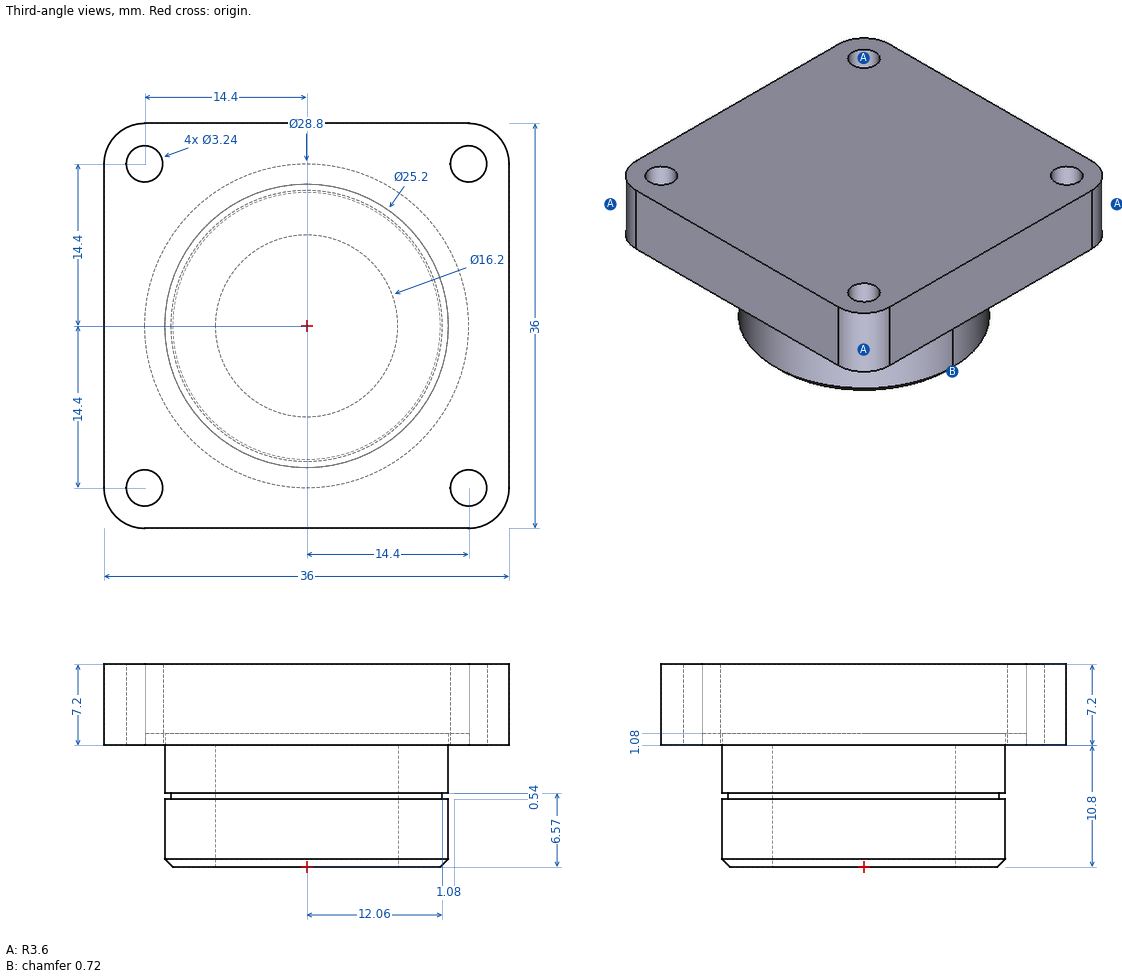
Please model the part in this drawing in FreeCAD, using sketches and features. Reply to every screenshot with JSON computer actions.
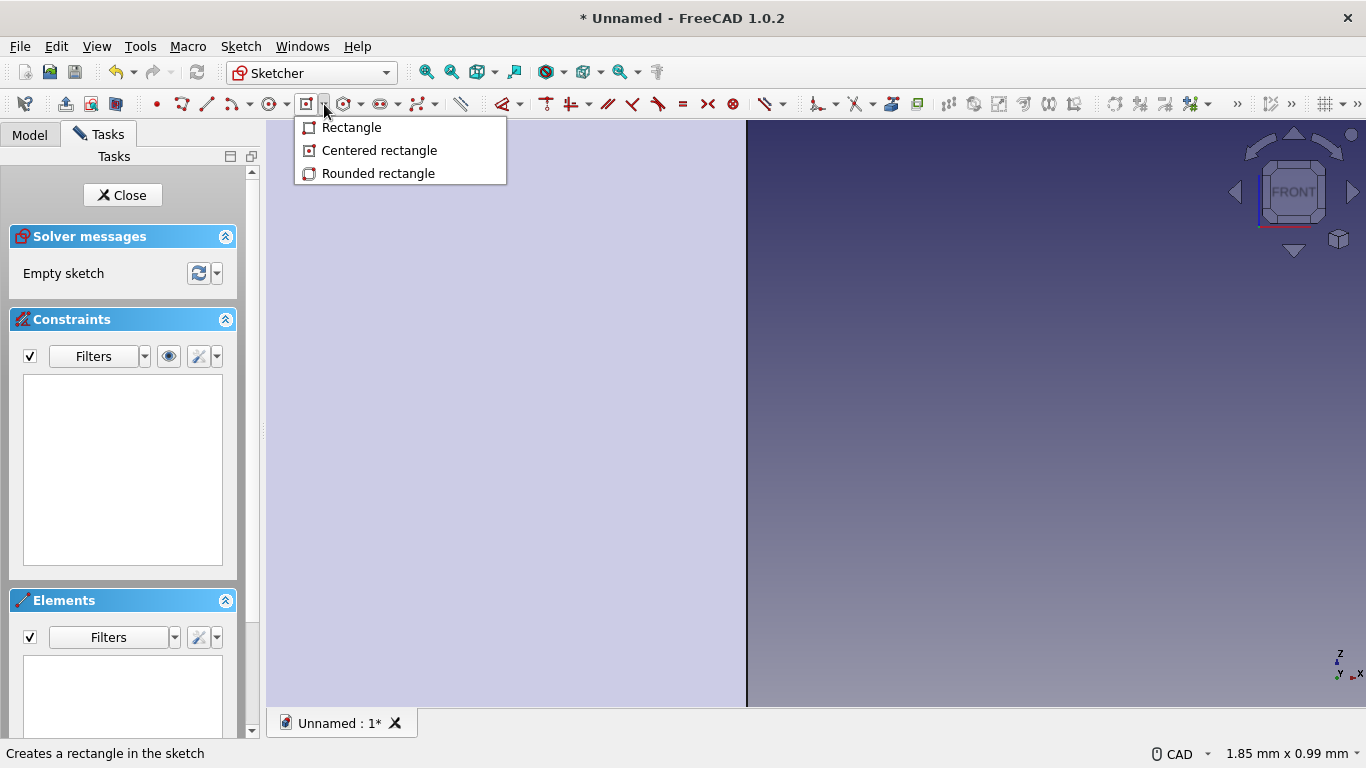
{"action": "left_click", "coordinate": [400, 128]}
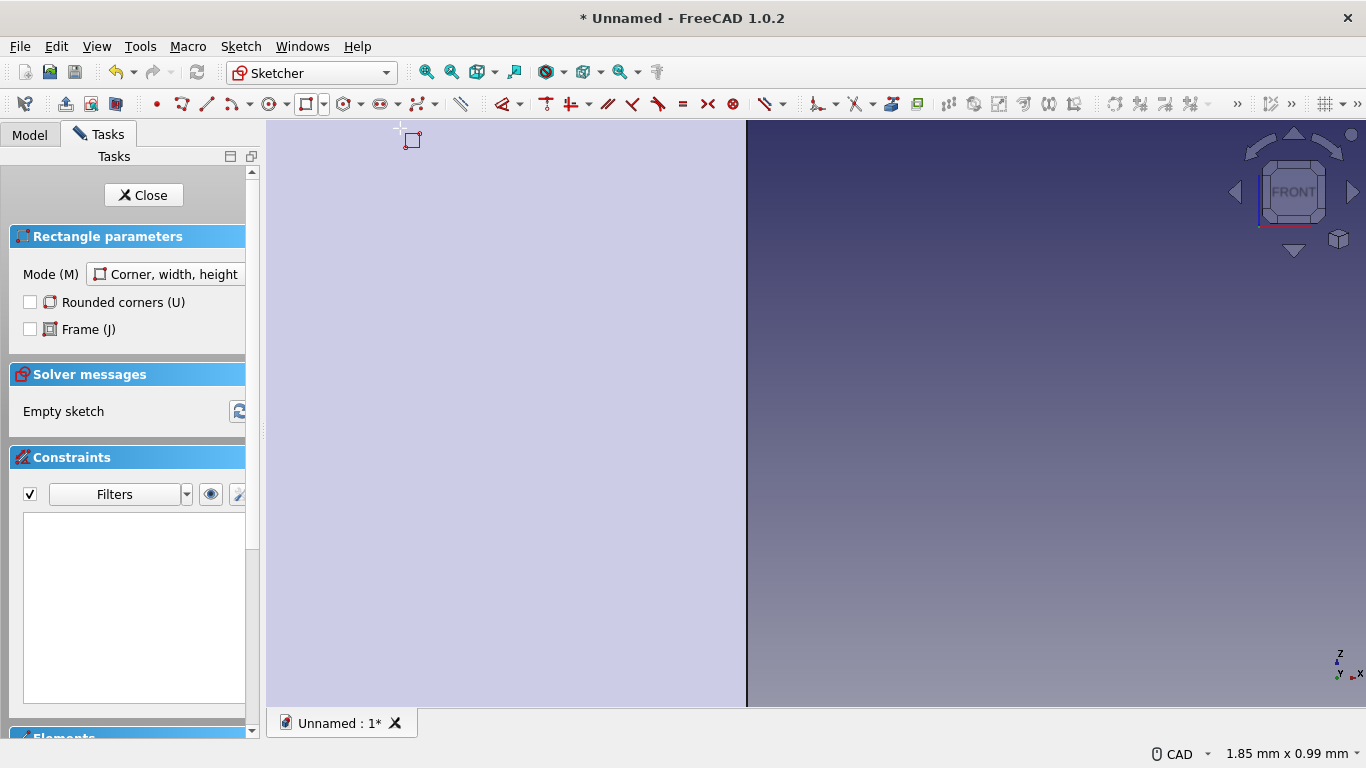
{"action": "left_click", "coordinate": [427, 252]}
{"action": "mouse_move", "coordinate": [1068, 572]}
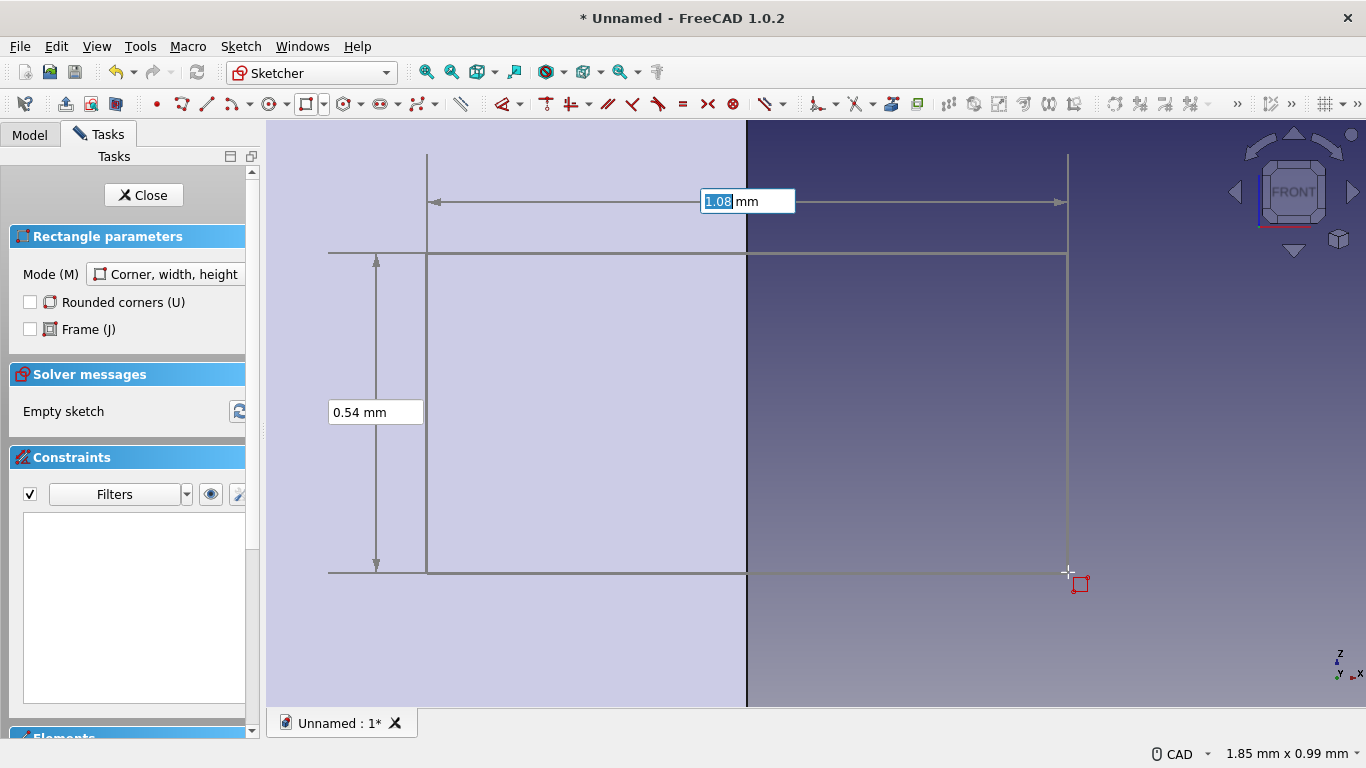
{"action": "type", "text": "1.08"}
{"action": "key", "text": "Tab"}
{"action": "type", "text": "0.54"}
{"action": "key", "text": "Return"}
{"action": "key", "text": "Escape"}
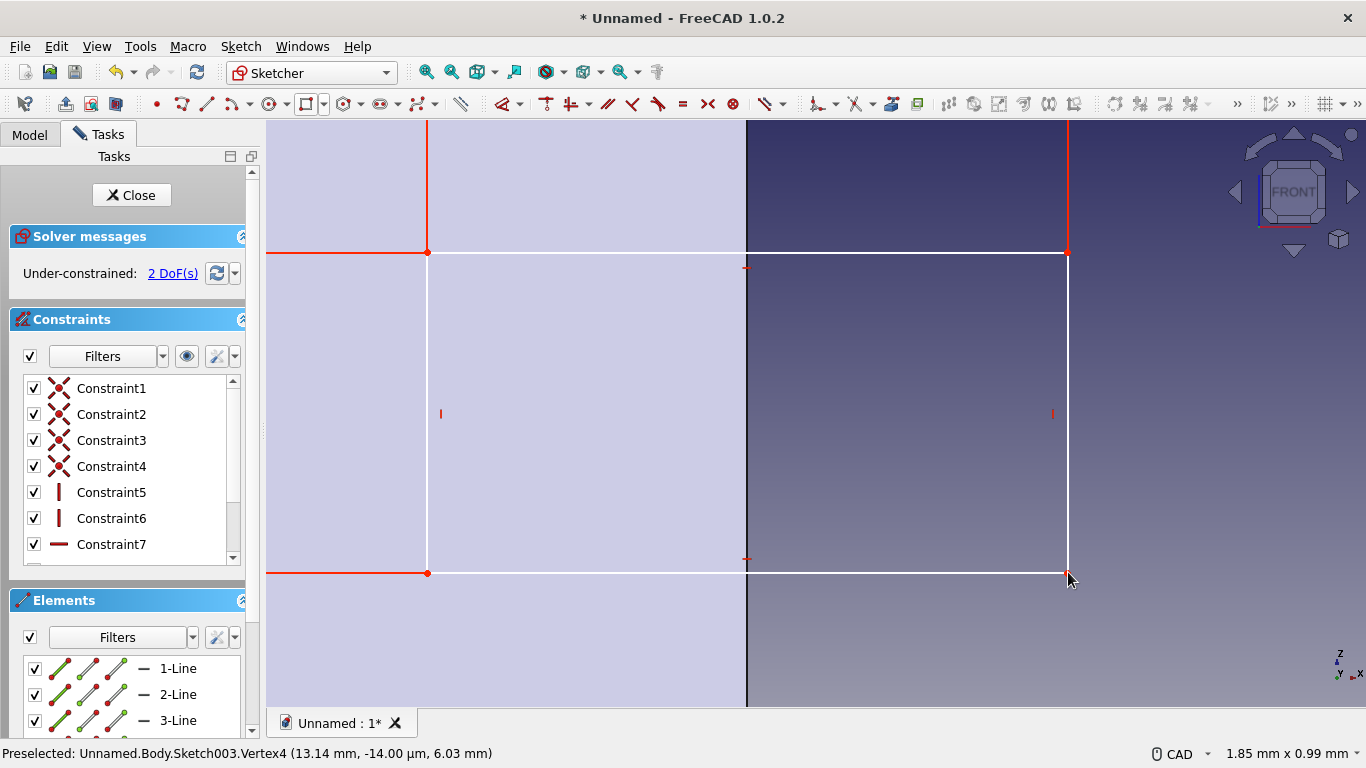
{"action": "left_click", "coordinate": [502, 104]}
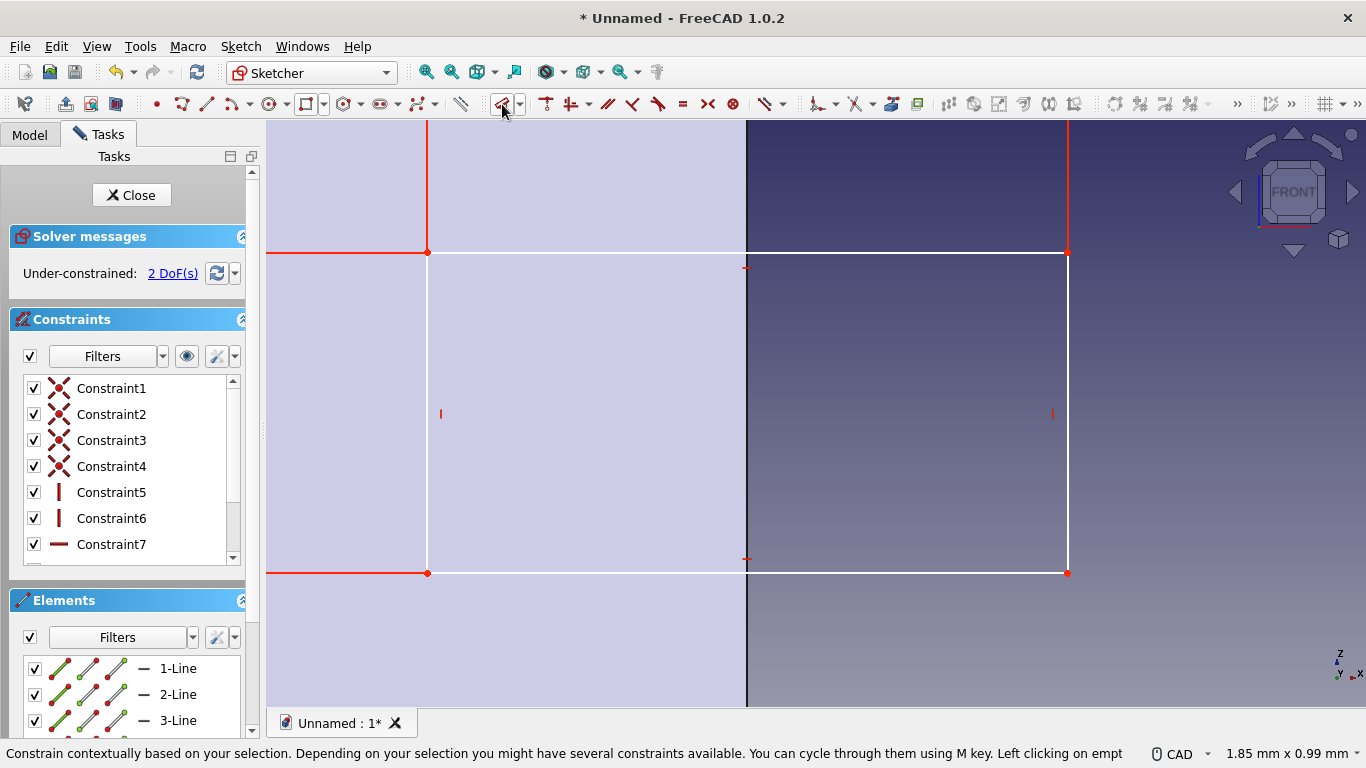
{"action": "left_click", "coordinate": [427, 253]}
{"action": "left_click", "coordinate": [461, 466]}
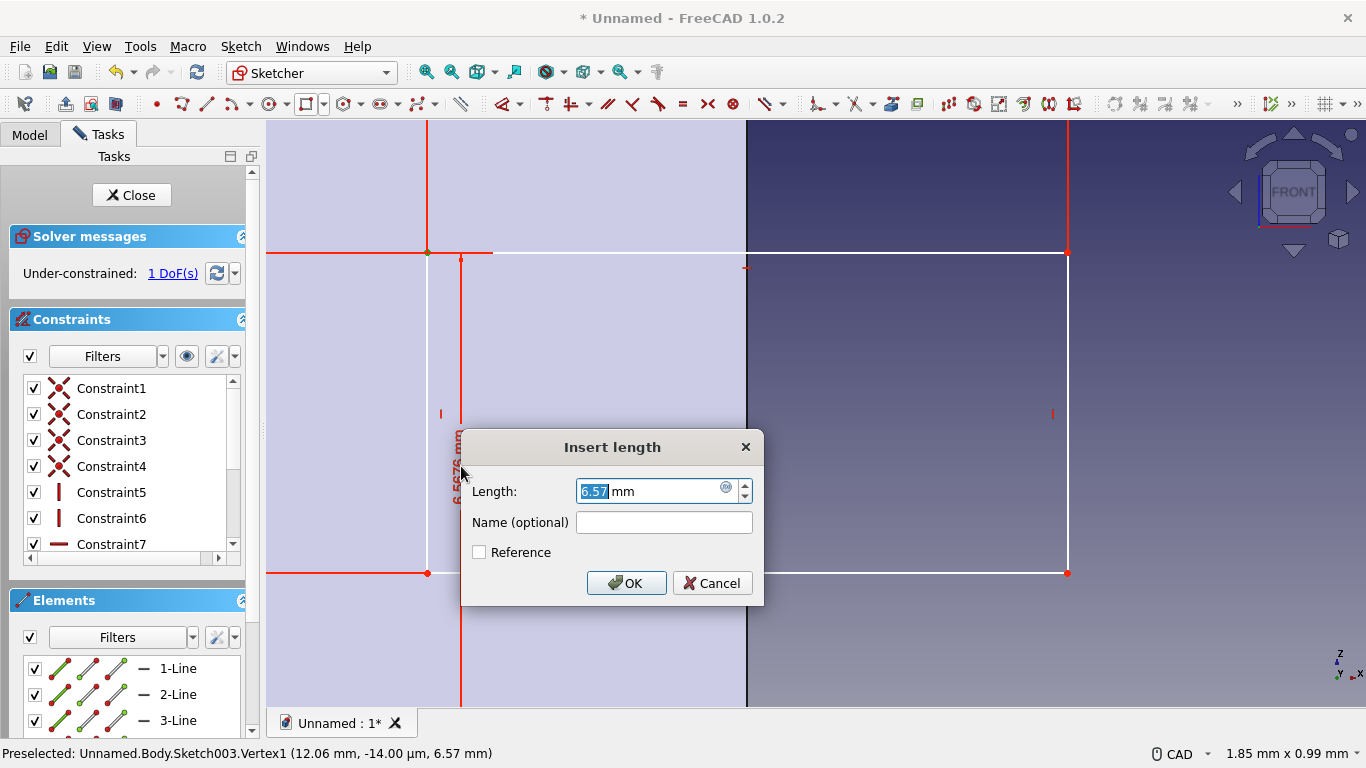
{"action": "type", "text": "6.57"}
{"action": "key", "text": "Return"}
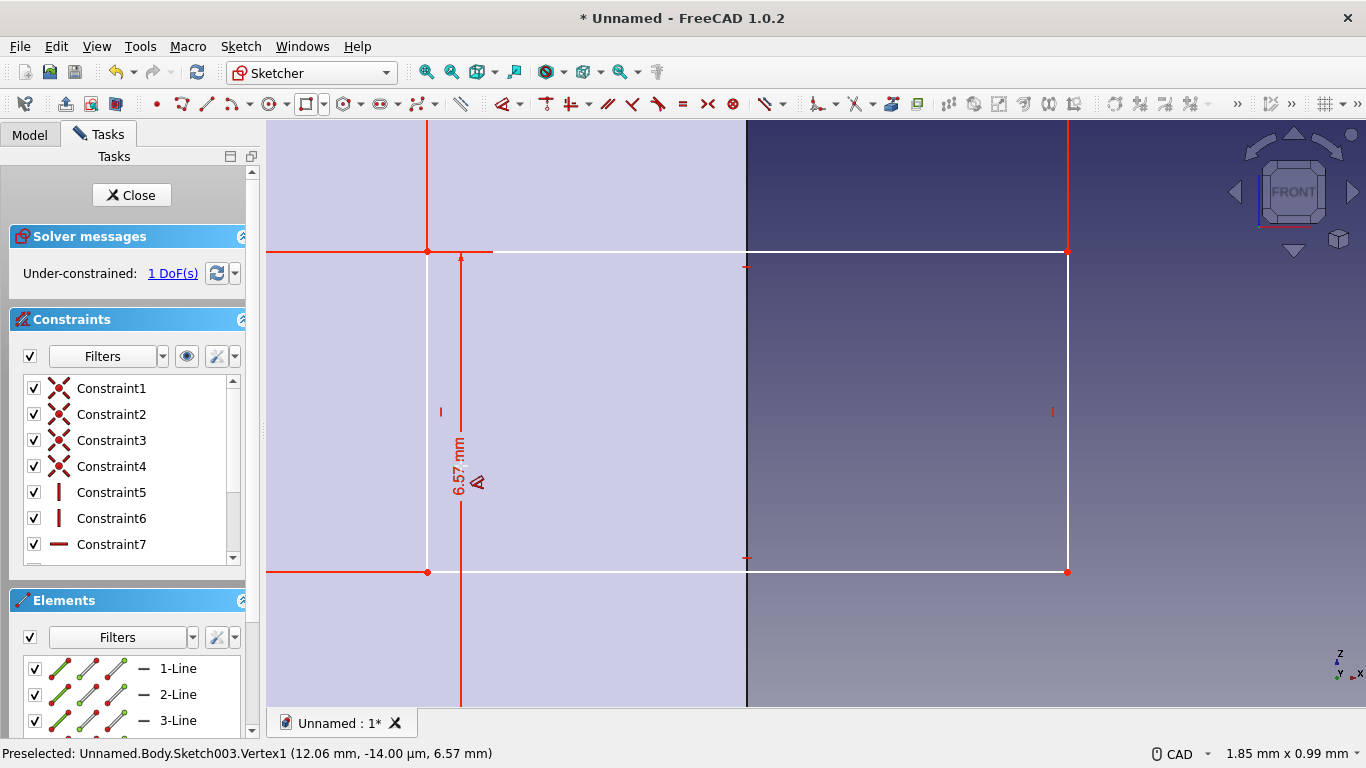
{"action": "left_click", "coordinate": [427, 252]}
{"action": "left_click", "coordinate": [361, 218]}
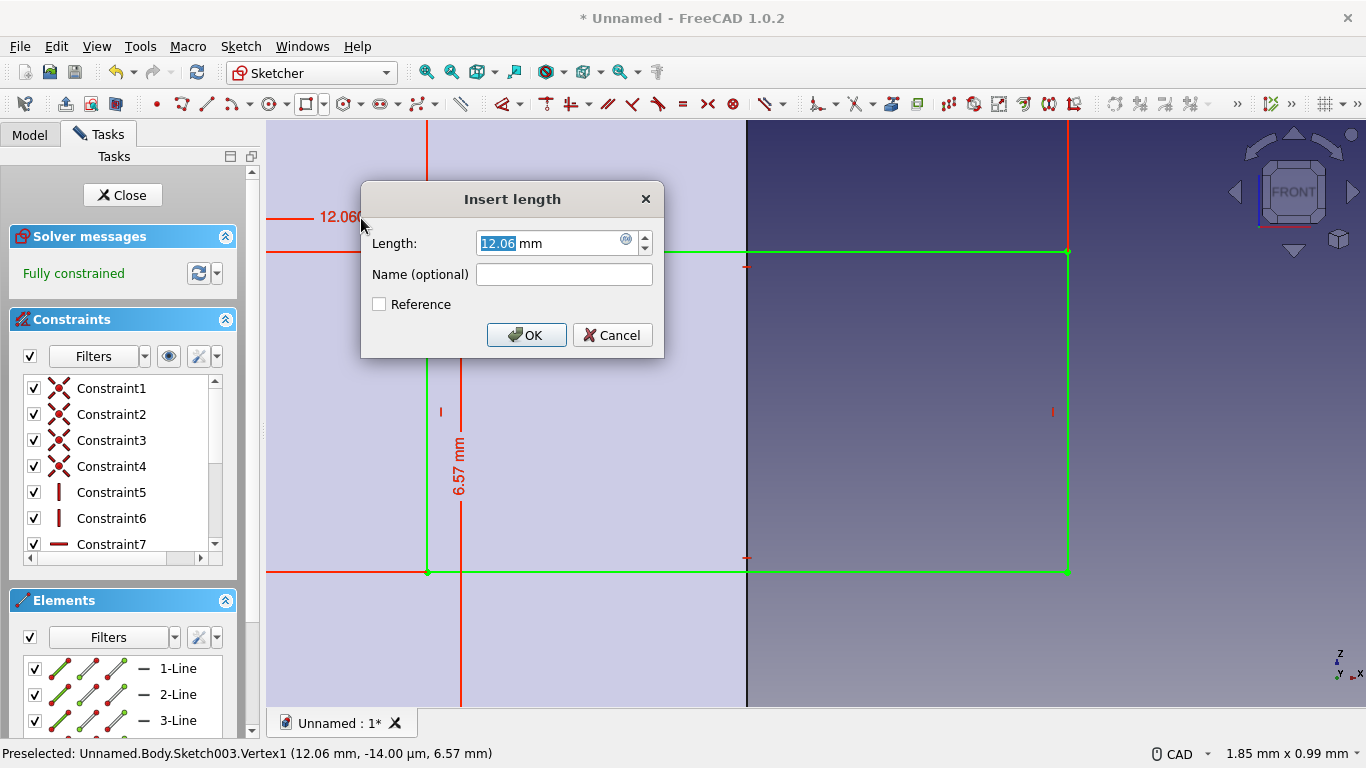
{"action": "type", "text": "12.06"}
{"action": "key", "text": "Return"}
{"action": "key", "text": "Escape"}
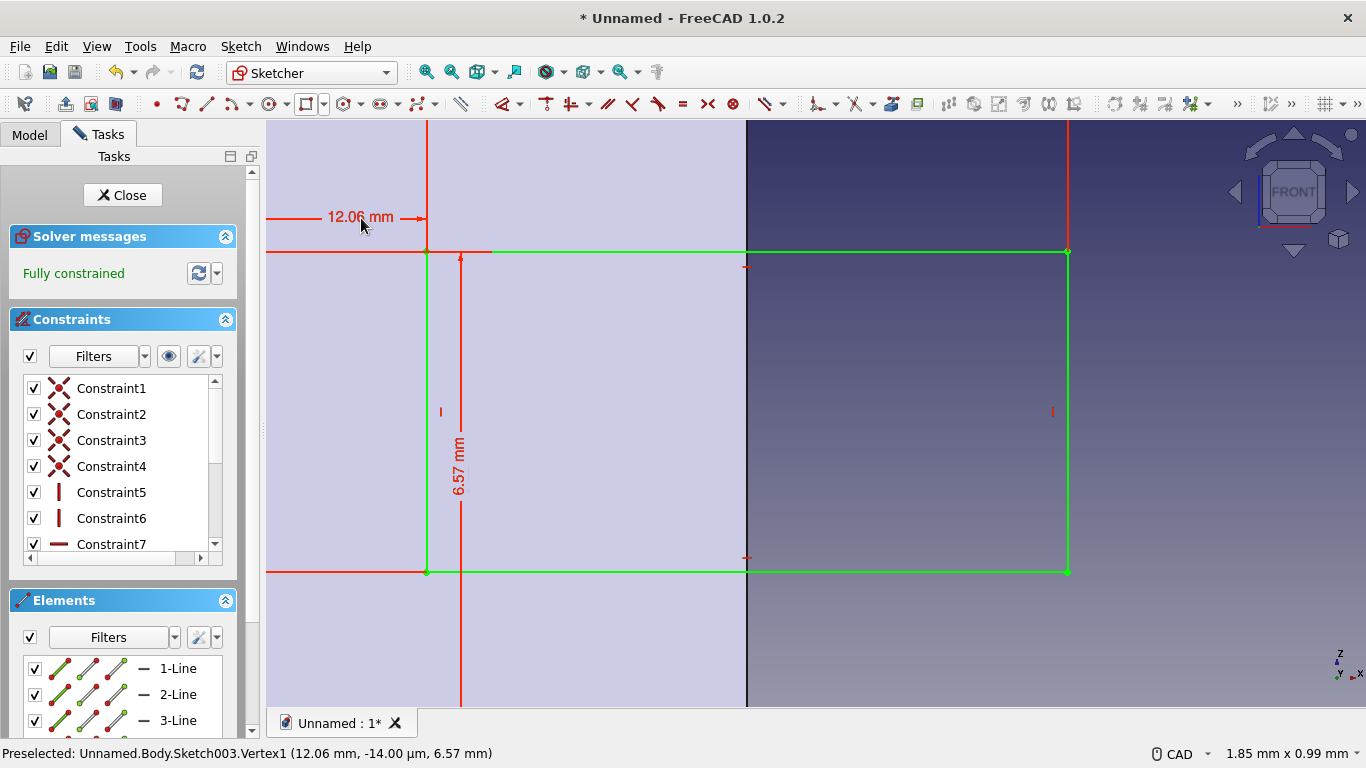
{"action": "left_click", "coordinate": [123, 195]}